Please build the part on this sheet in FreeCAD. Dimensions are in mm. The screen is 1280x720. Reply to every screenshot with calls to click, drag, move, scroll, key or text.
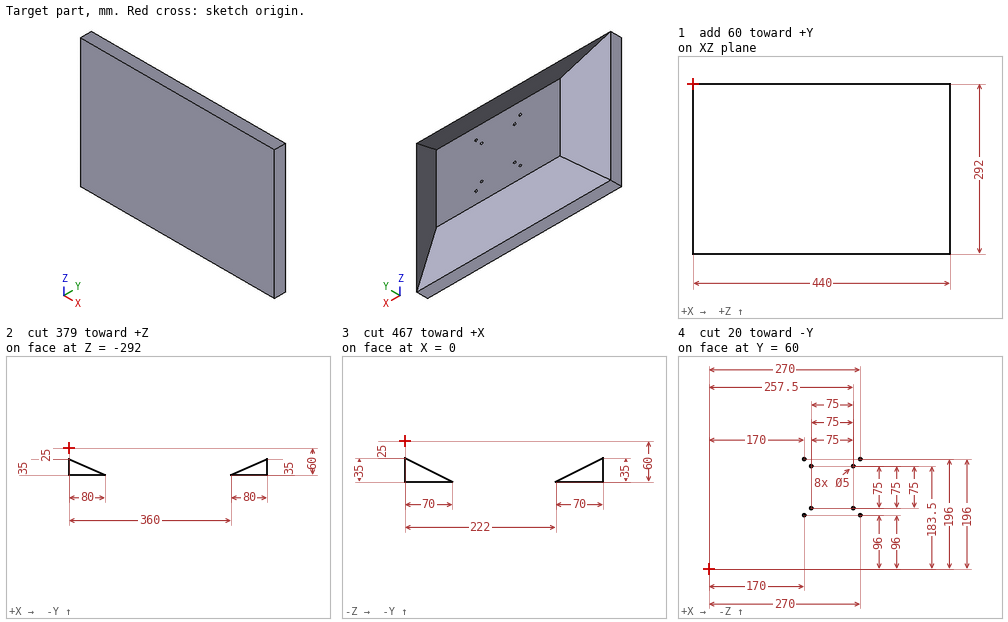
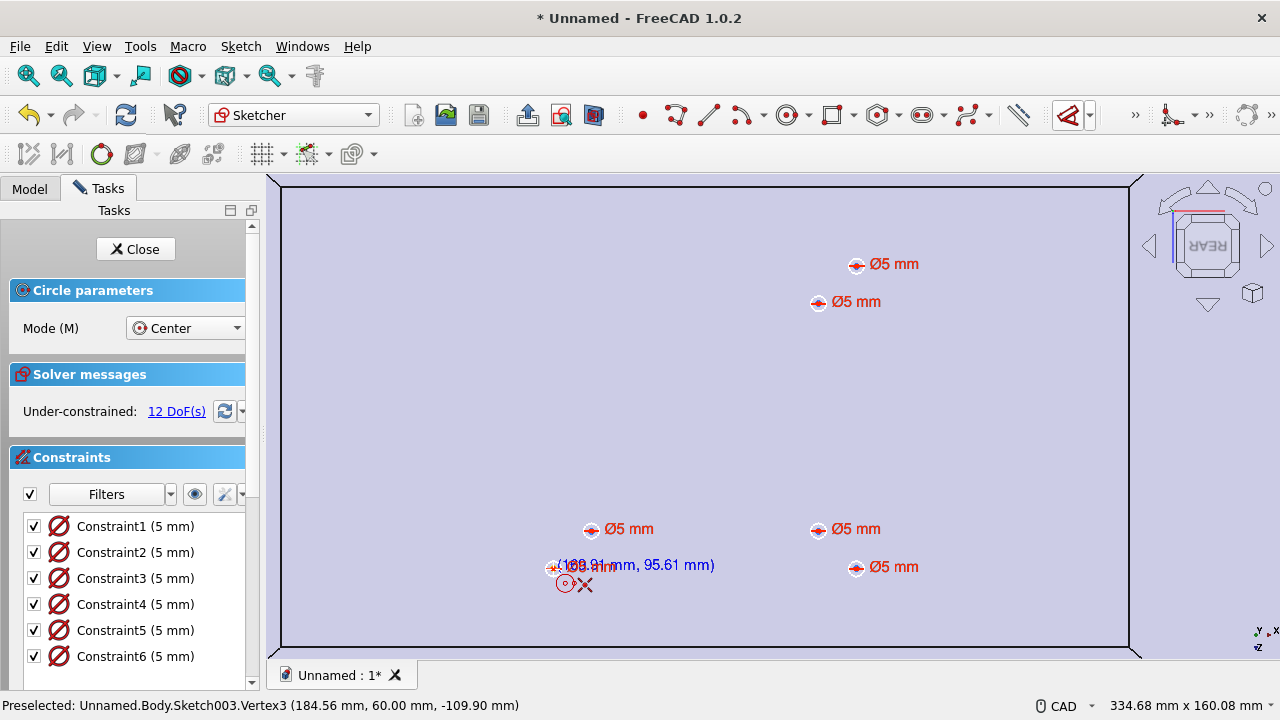
scroll(553, 266, up, 6)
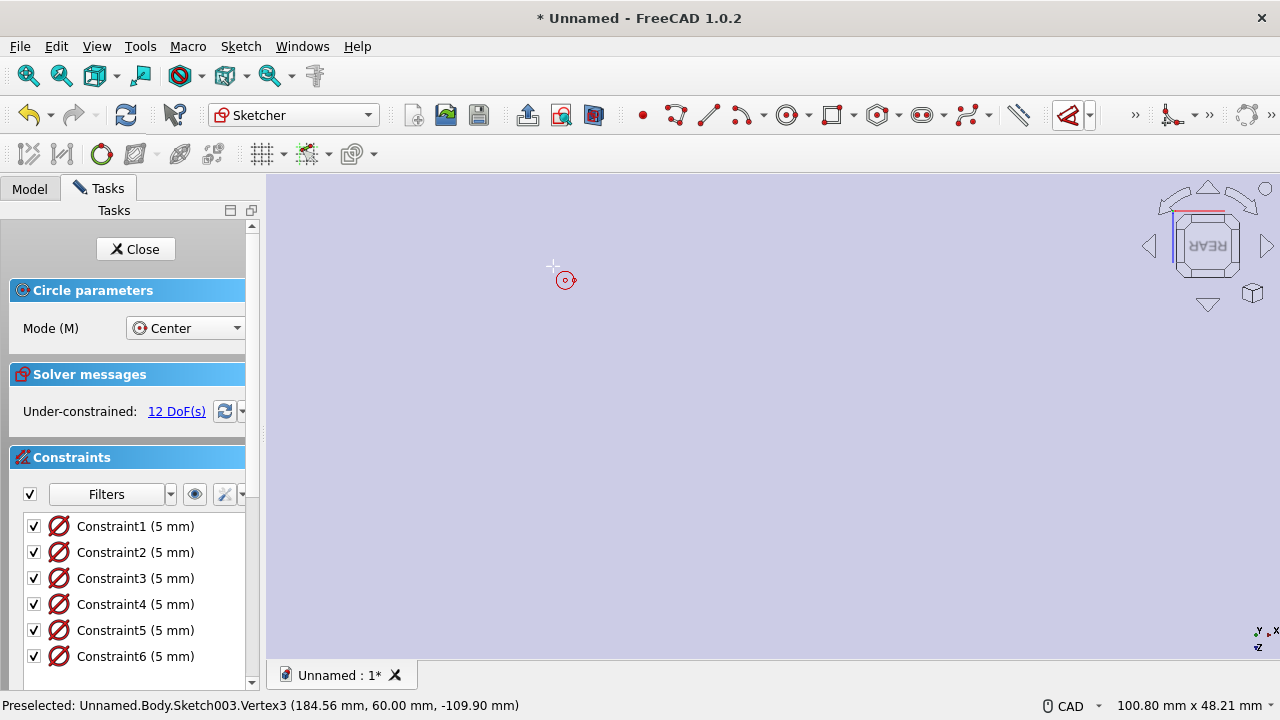
click(554, 265)
move(572, 247)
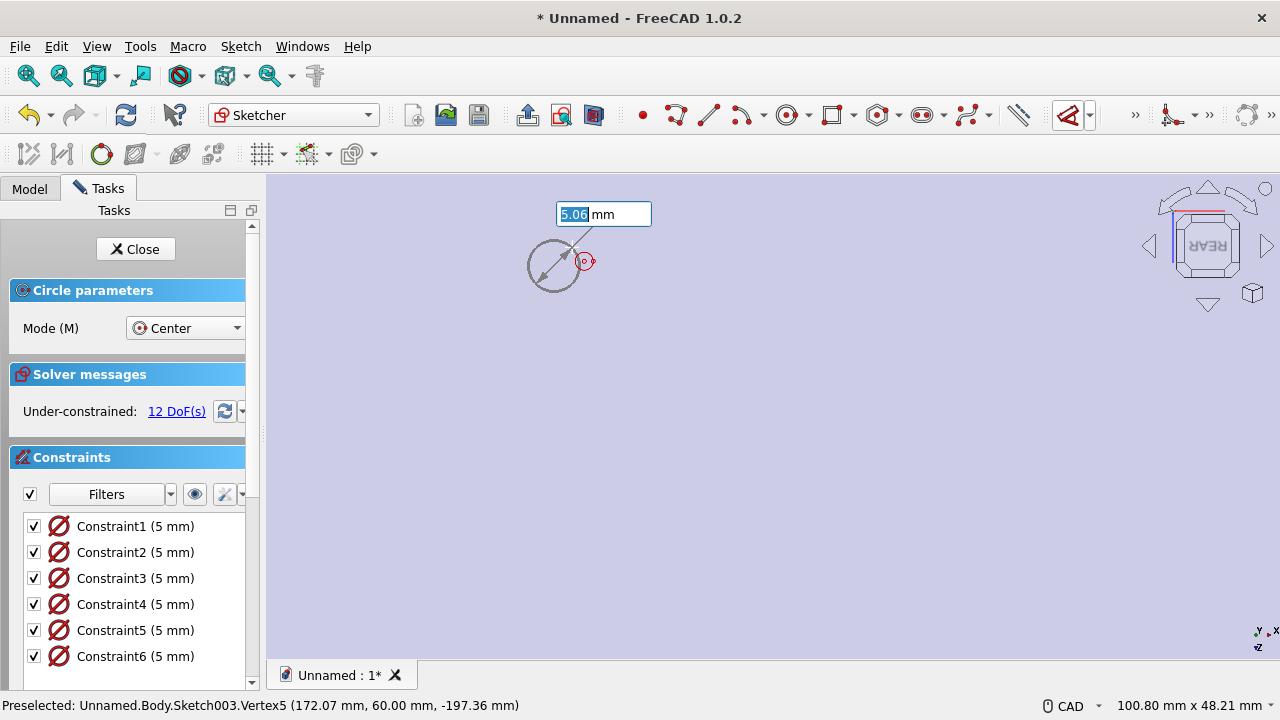
text(5)
key(Return)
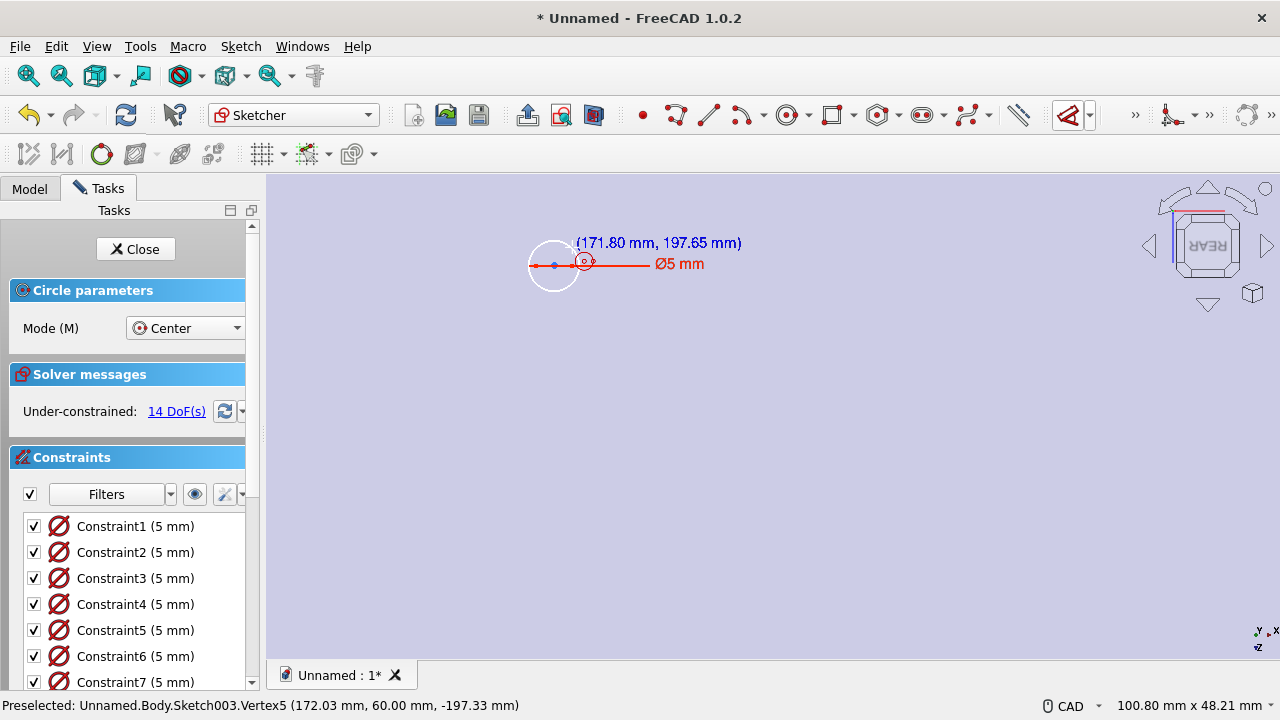
click(680, 390)
move(697, 373)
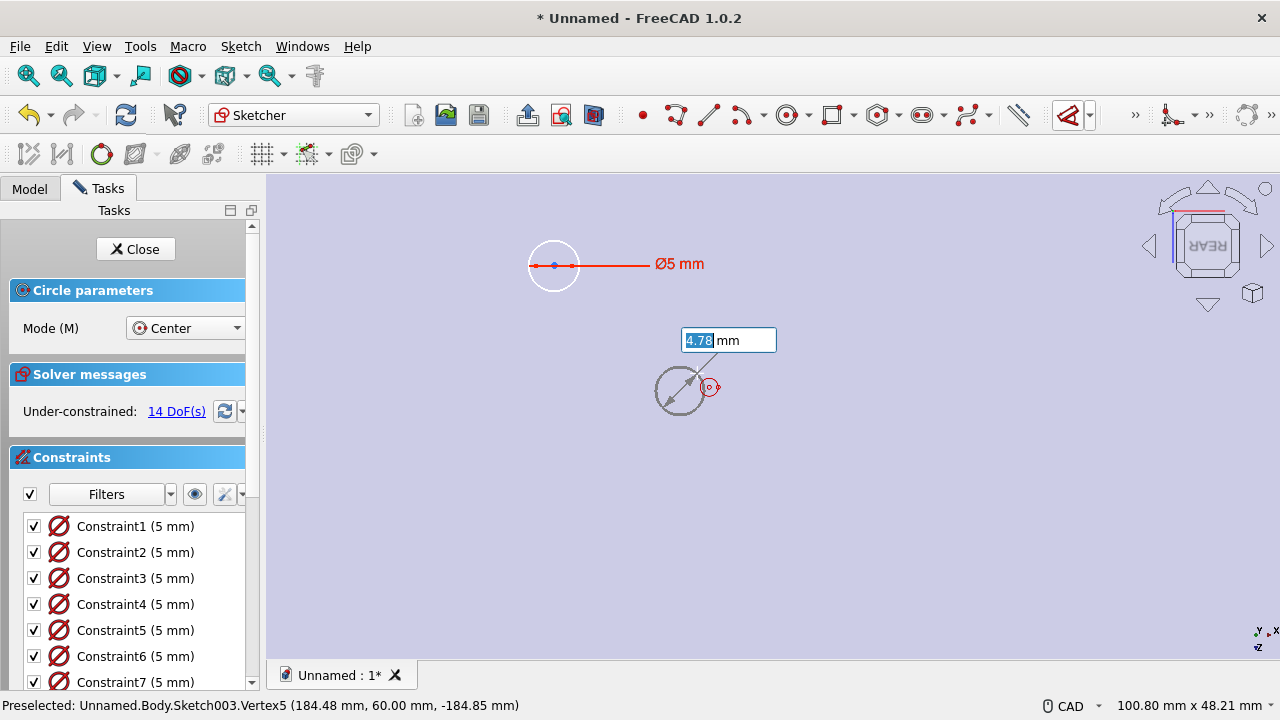
text(5)
key(Return)
key(Escape)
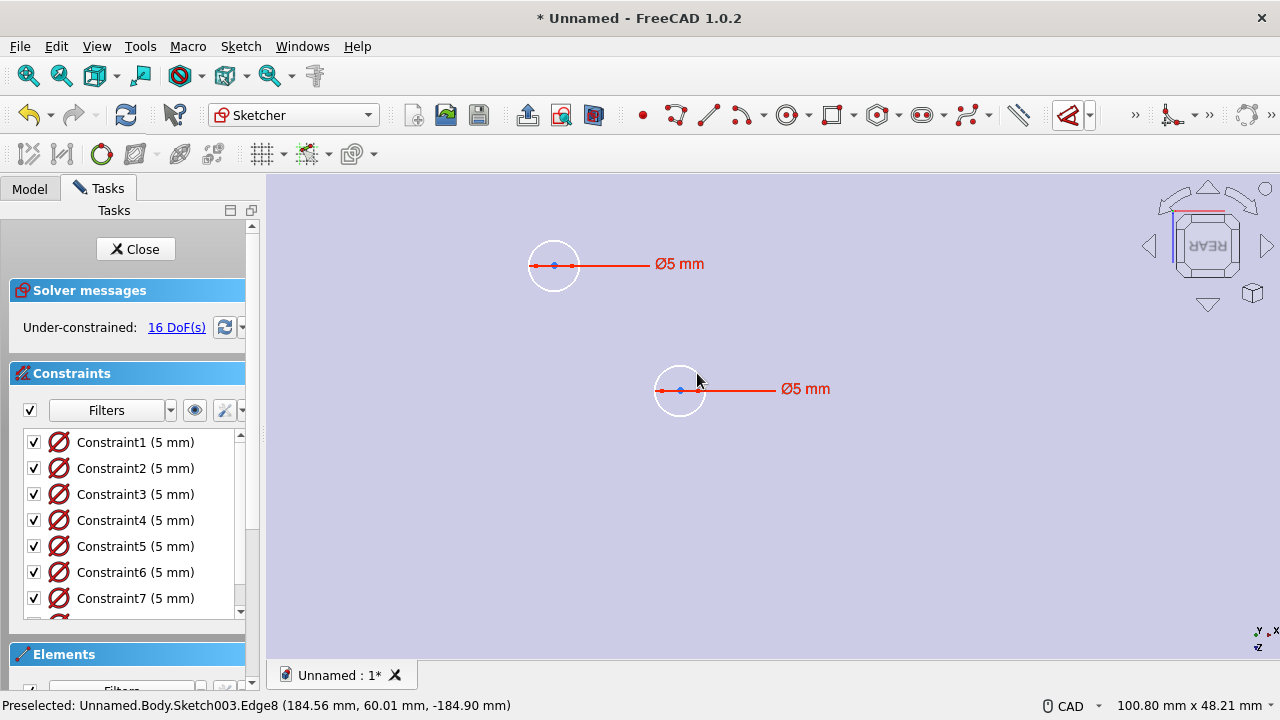
scroll(553, 265, down, 6)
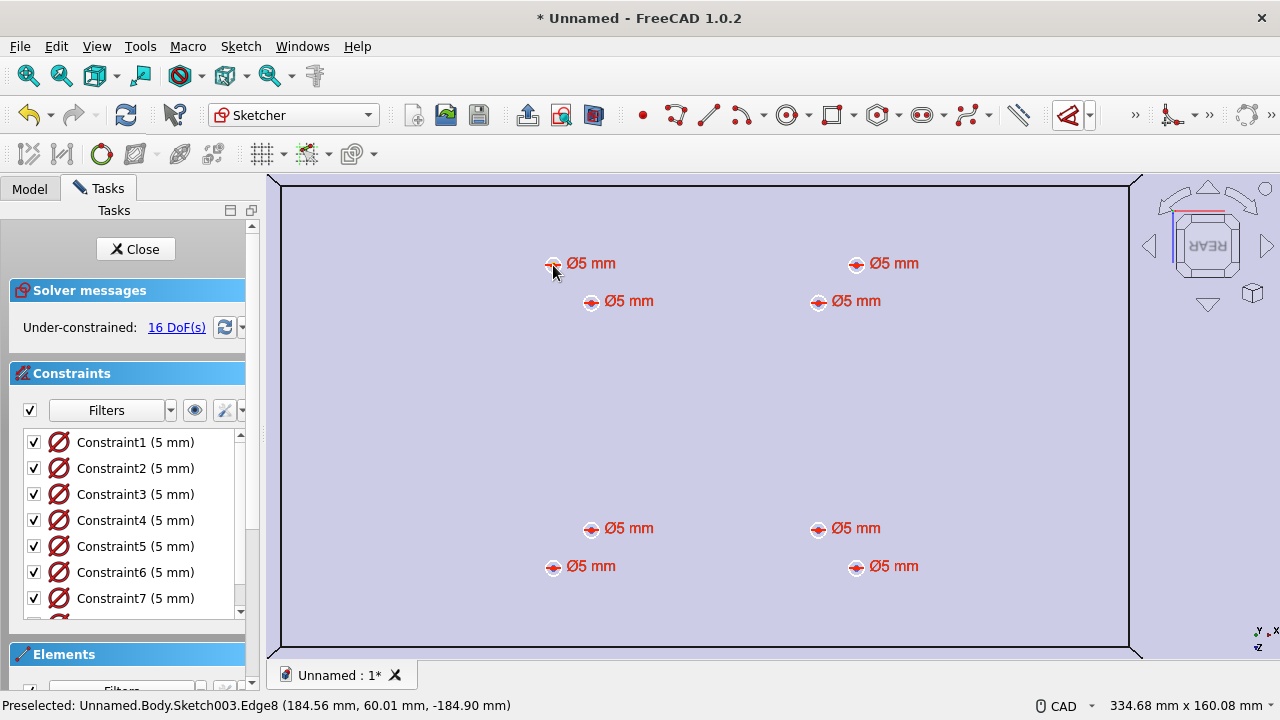
click(856, 568)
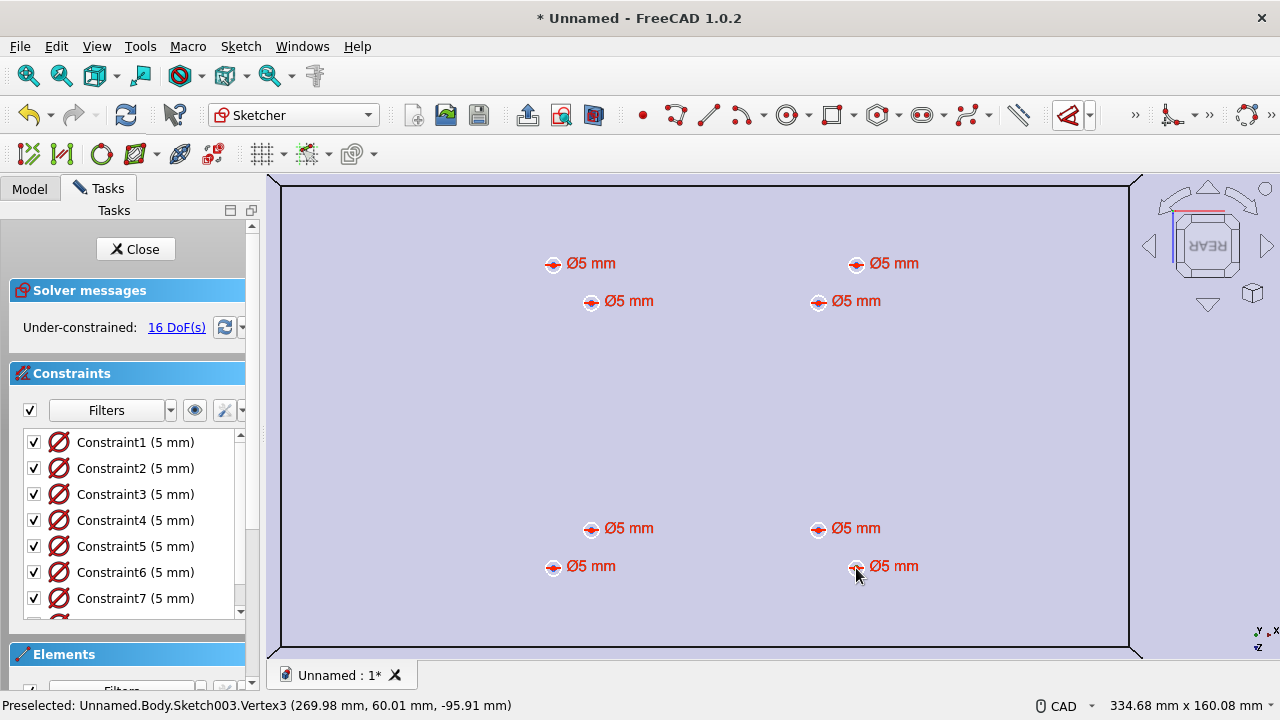
key(i)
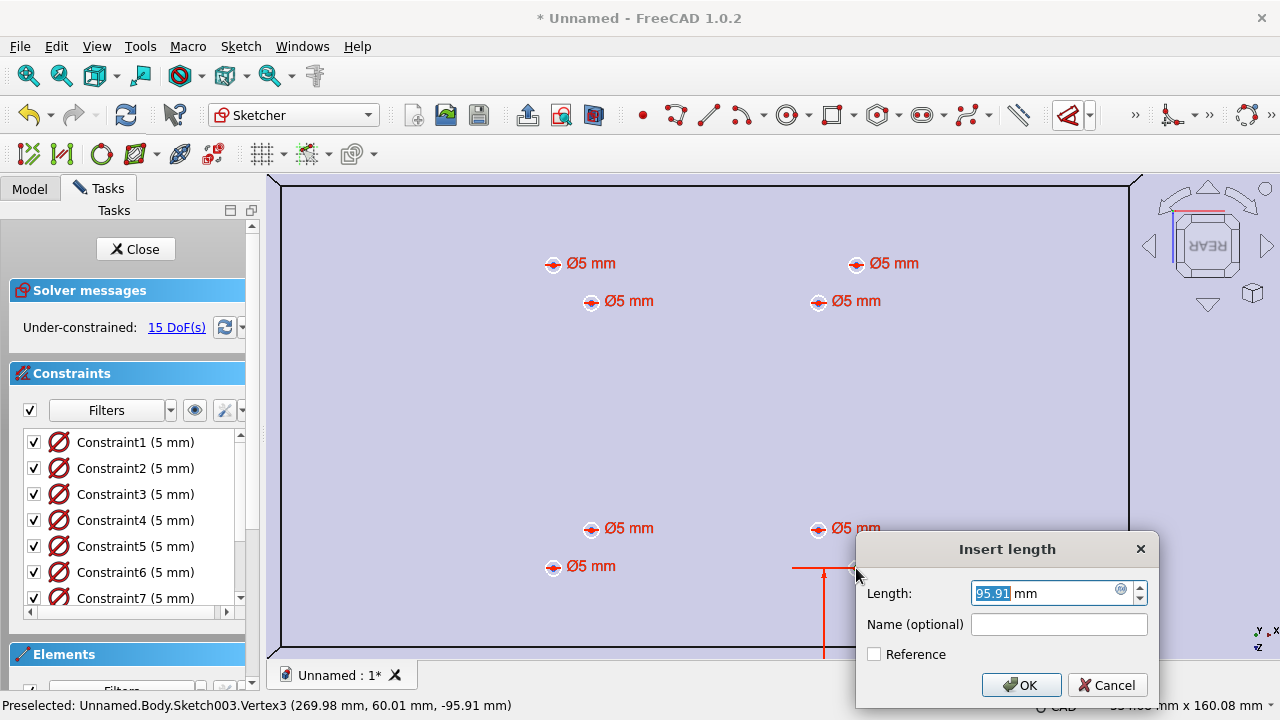
text(96)
key(Return)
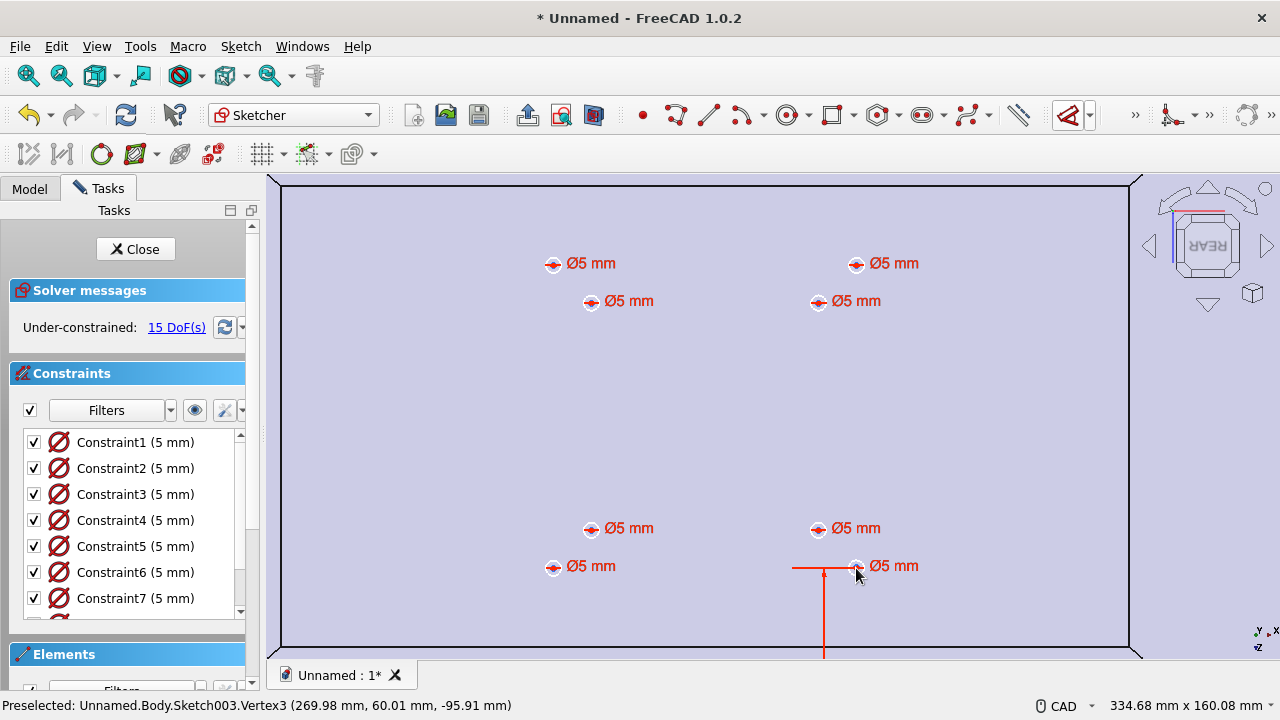
click(553, 568)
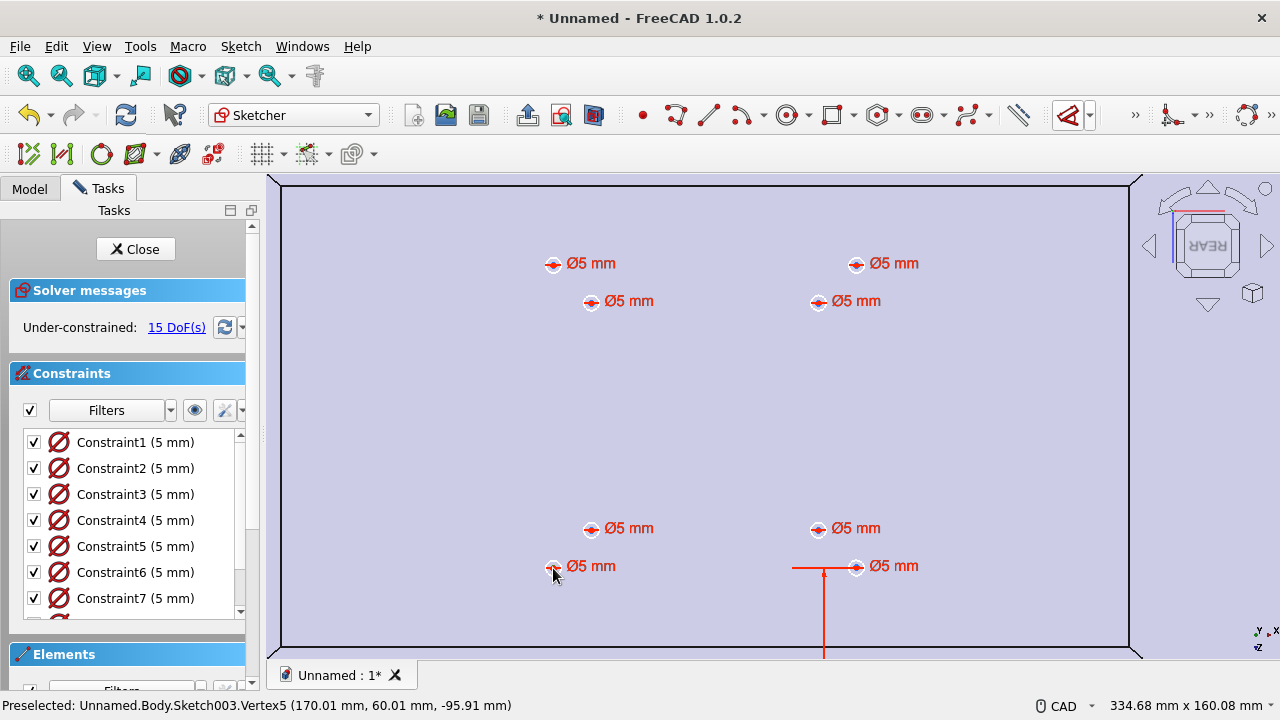
key(i)